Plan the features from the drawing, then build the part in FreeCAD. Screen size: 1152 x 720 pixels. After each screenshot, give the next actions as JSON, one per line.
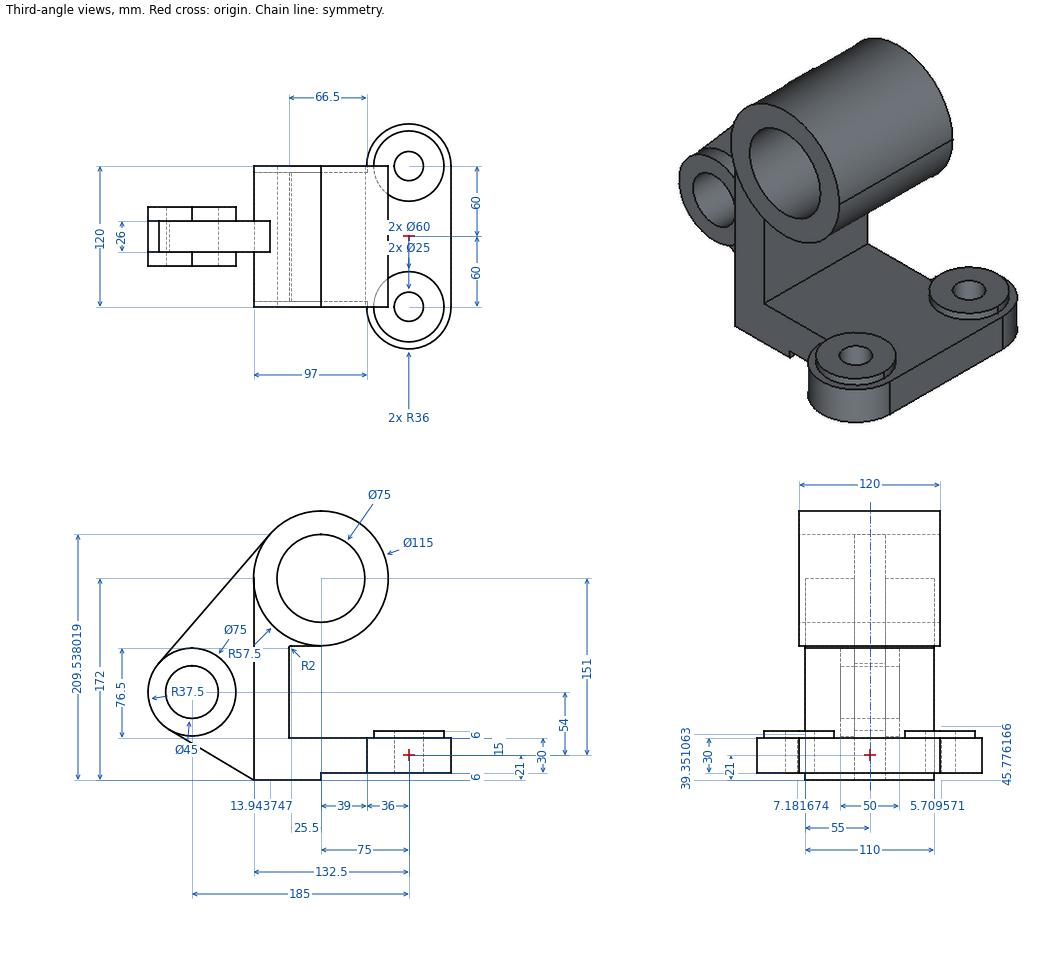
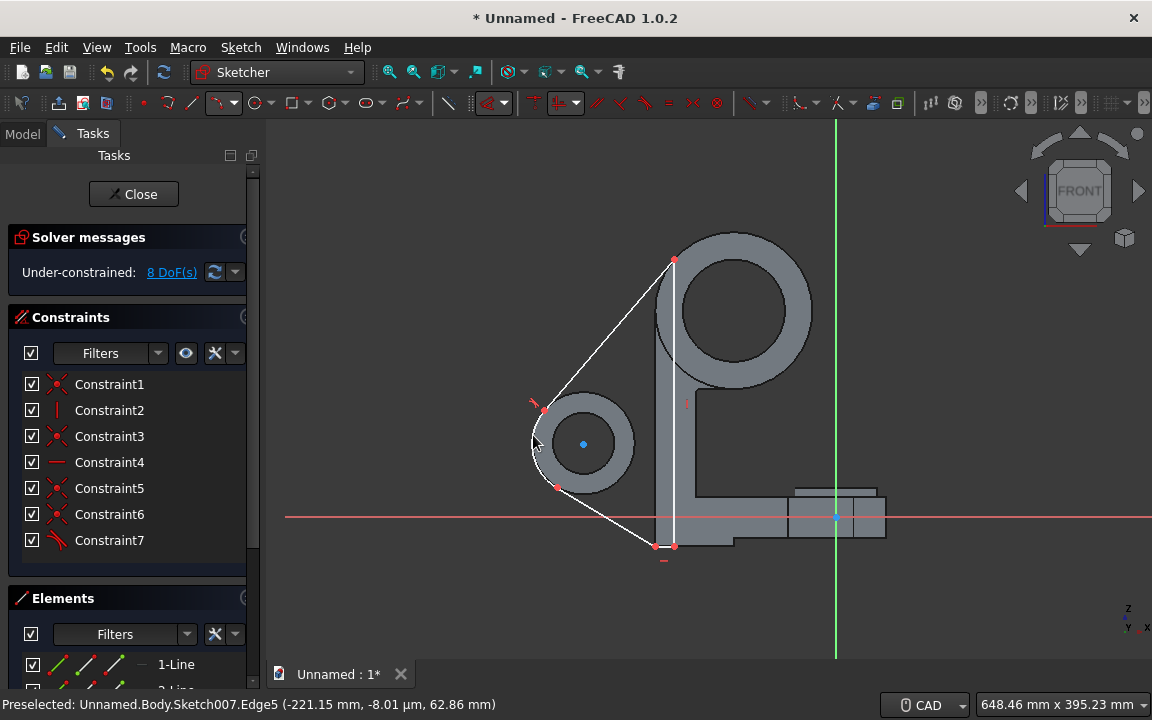
{"action": "left_click", "coordinate": [626, 529]}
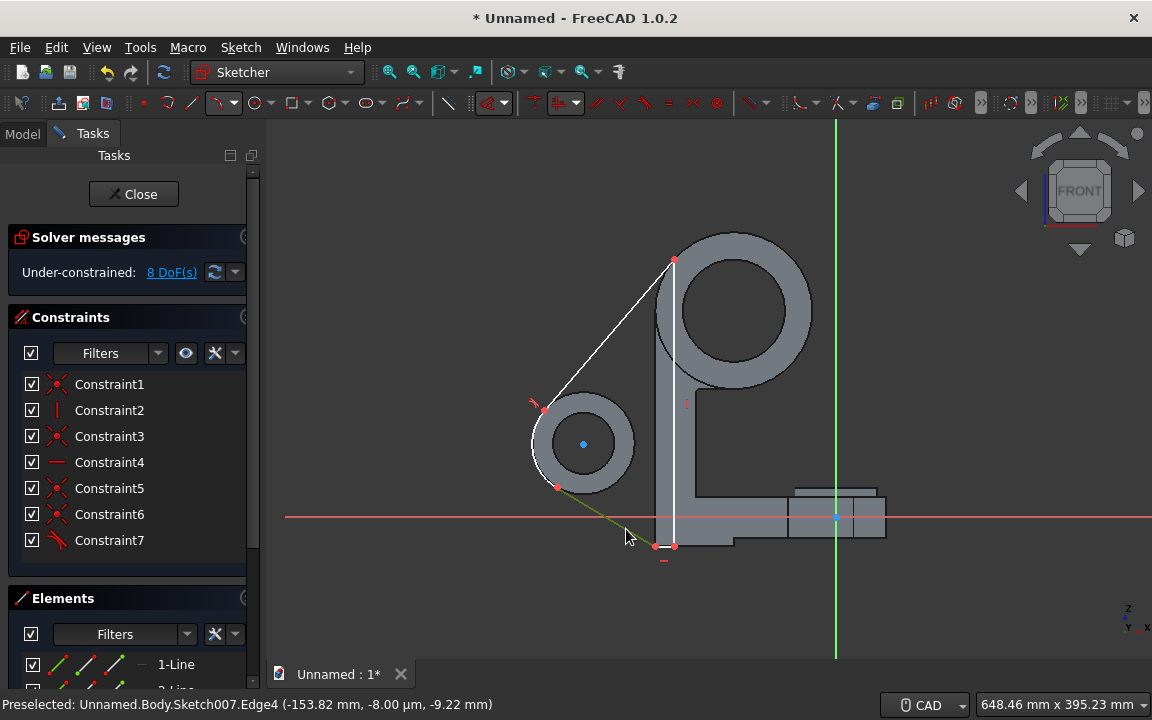
{"action": "left_click", "coordinate": [533, 435]}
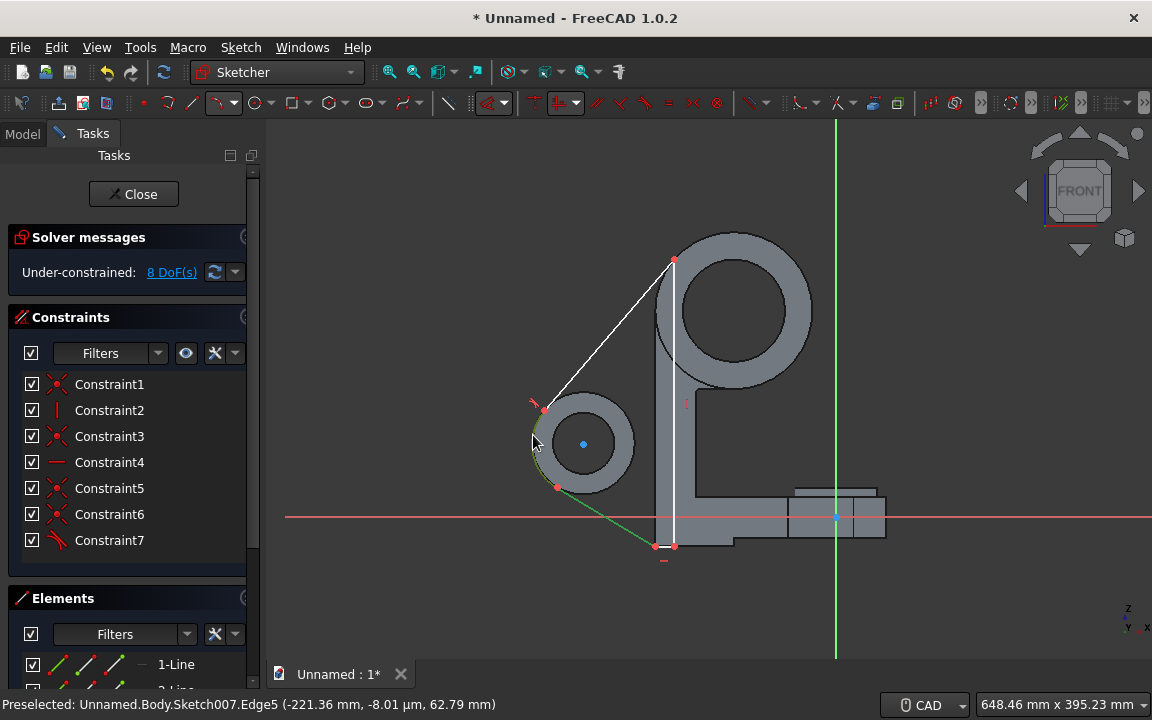
{"action": "left_click", "coordinate": [646, 104]}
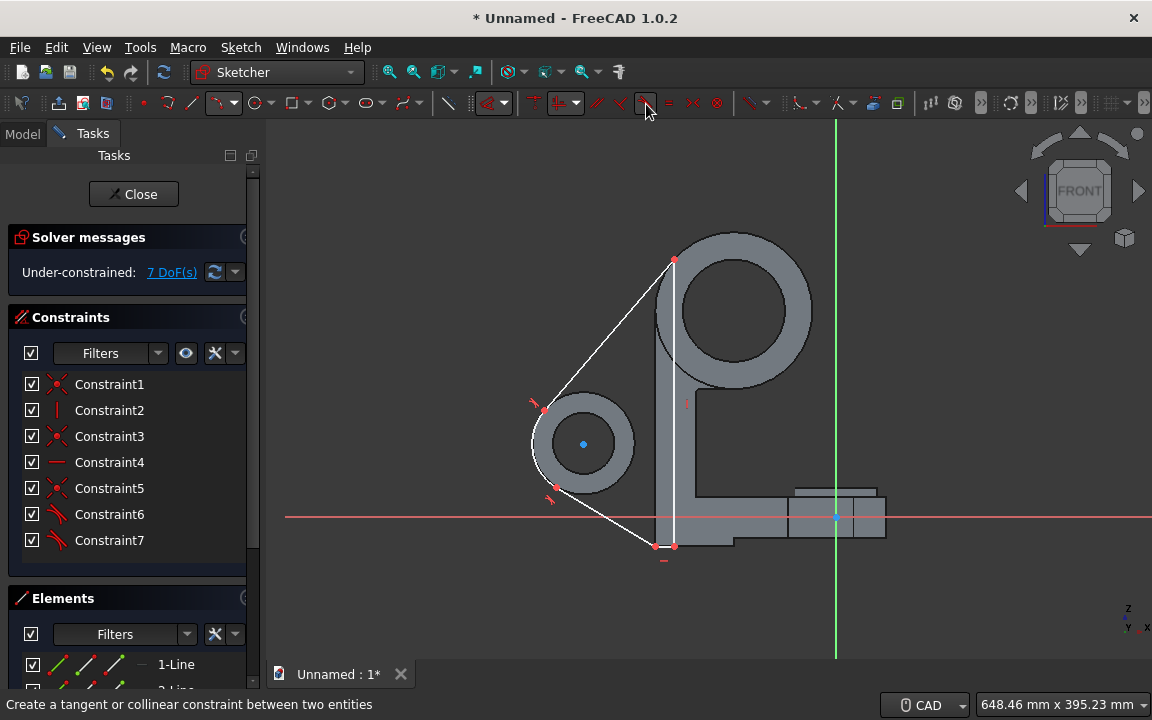
{"action": "left_click", "coordinate": [533, 435]}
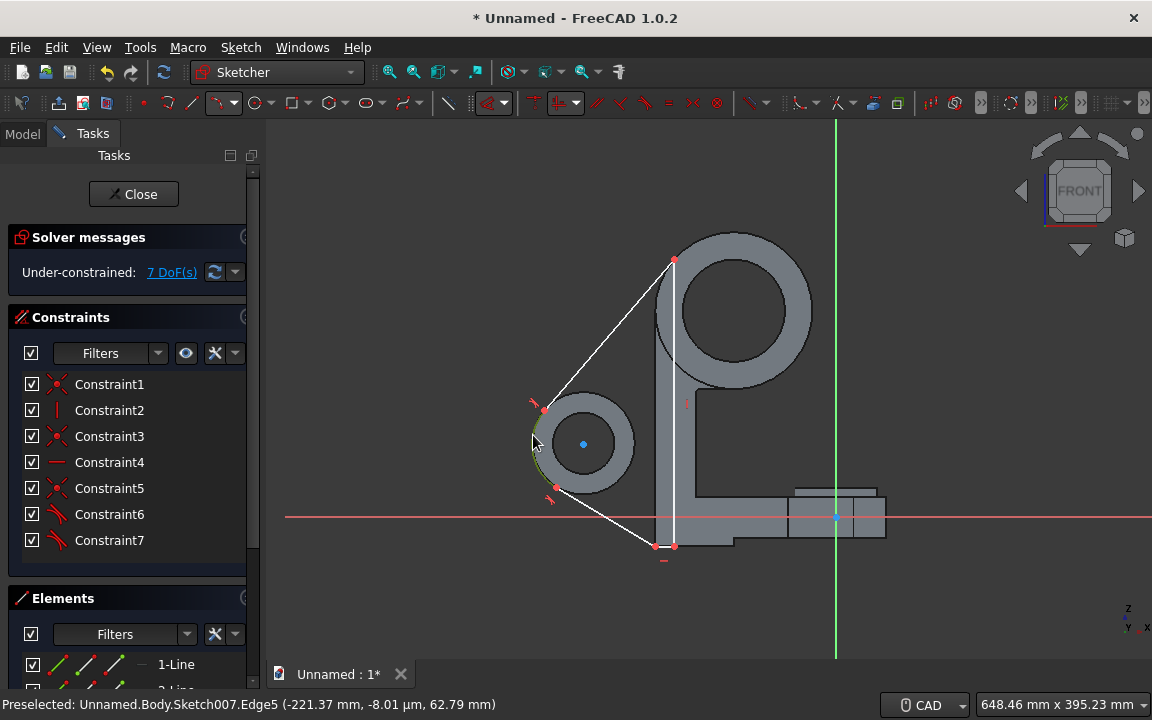
{"action": "key", "text": "k r"}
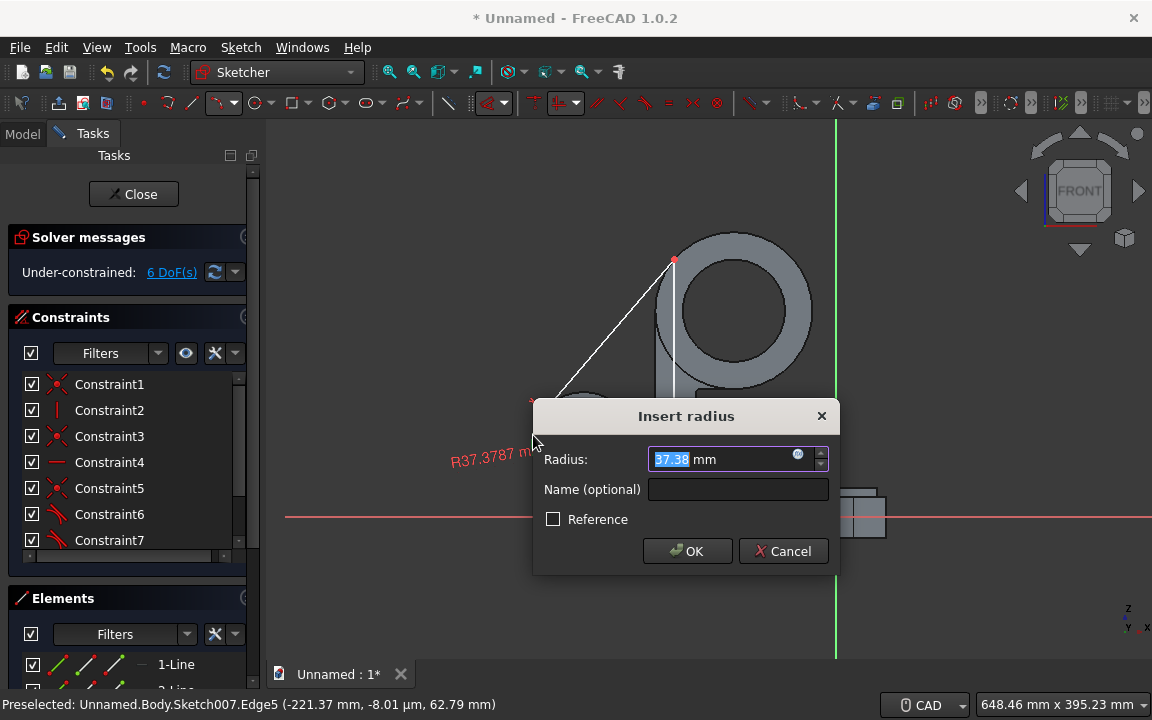
{"action": "type", "text": "37.5"}
{"action": "key", "text": "Return"}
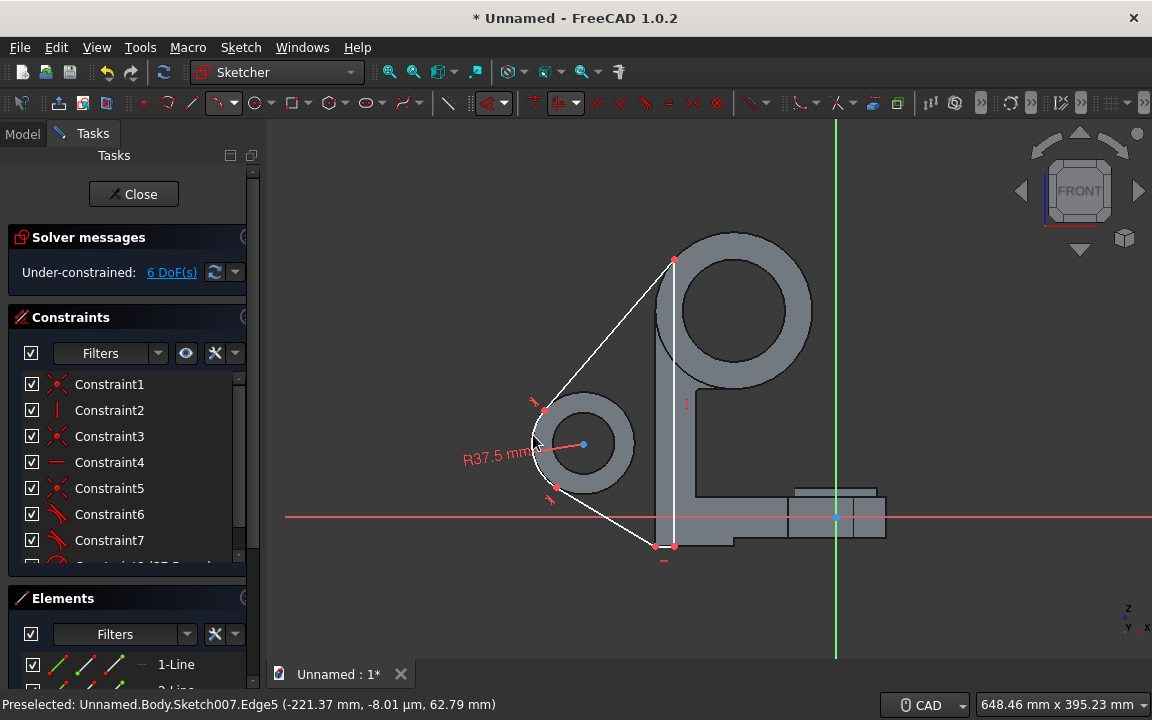
{"action": "scroll", "coordinate": [674, 547], "scroll_direction": "up", "scroll_amount": 2}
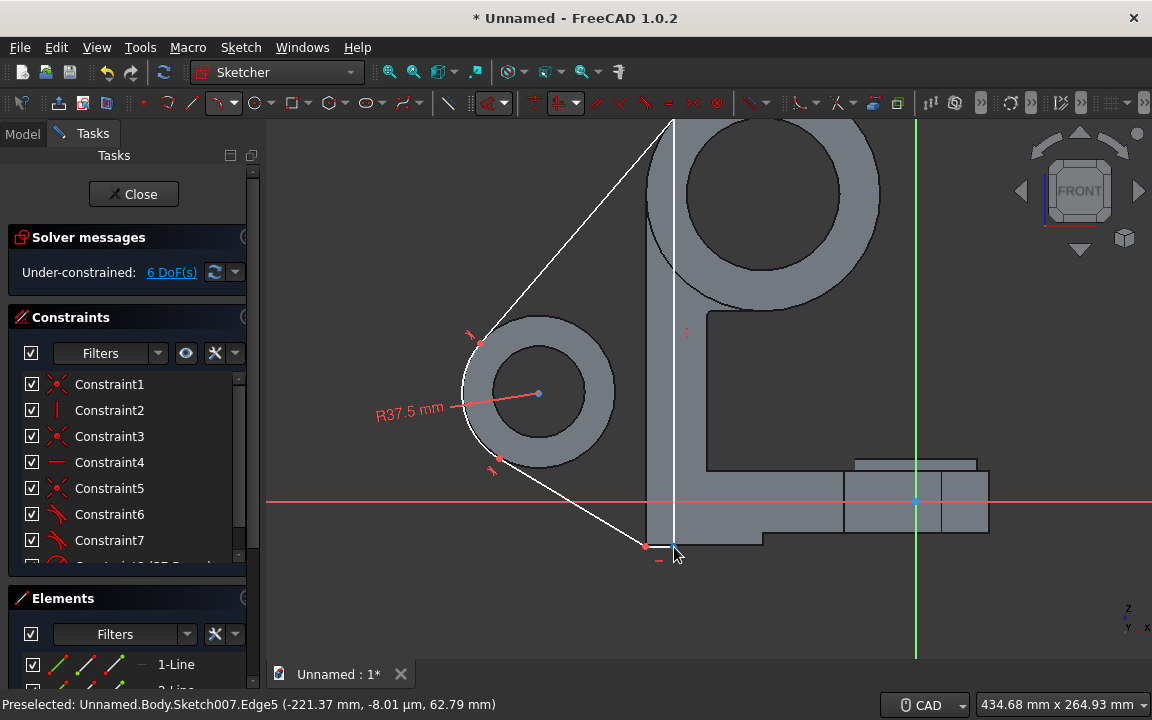
{"action": "left_click", "coordinate": [674, 547]}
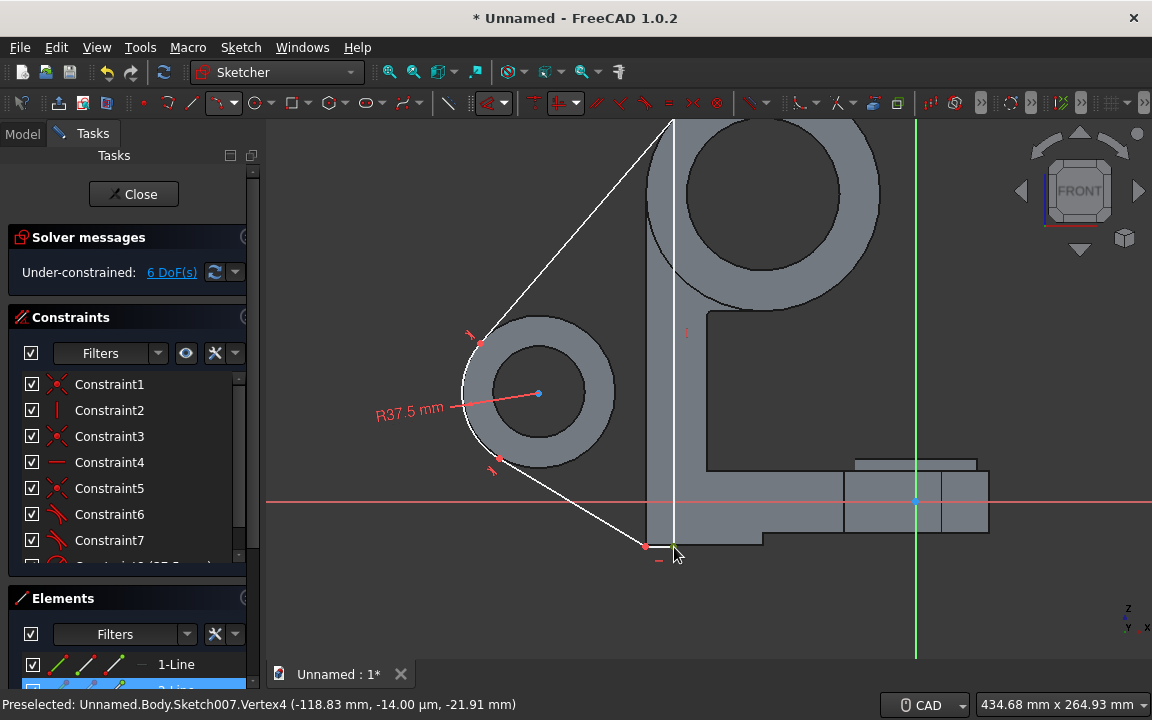
{"action": "left_click", "coordinate": [506, 104]}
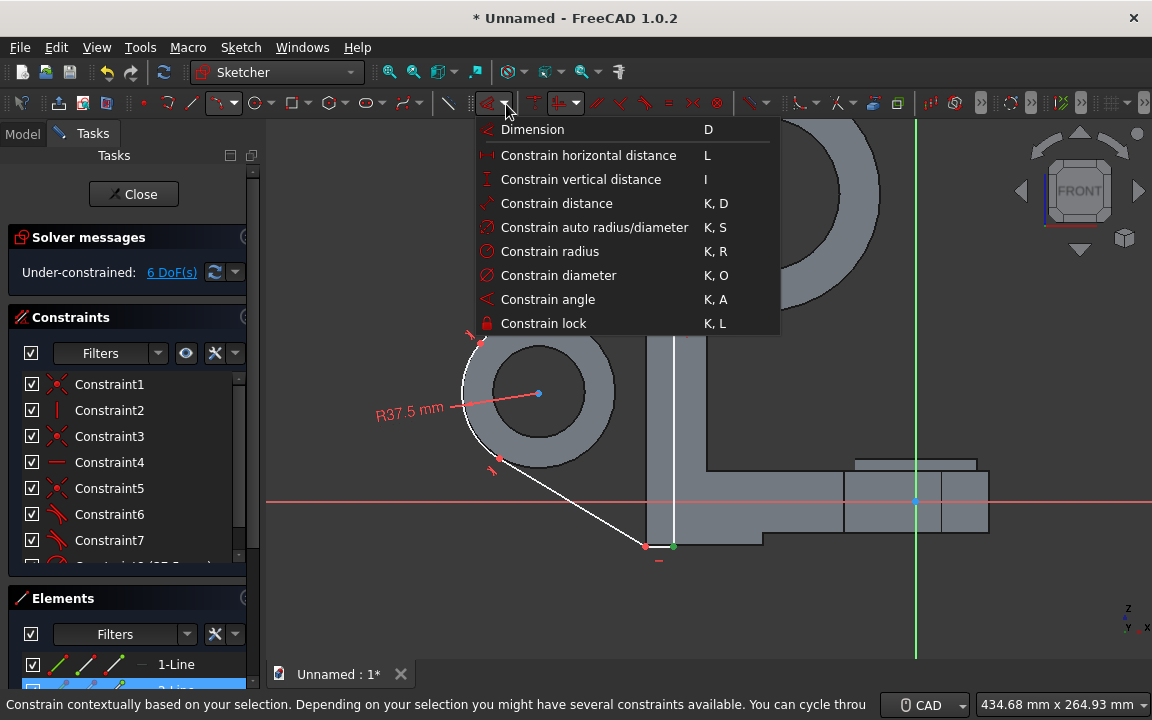
{"action": "left_click", "coordinate": [628, 179]}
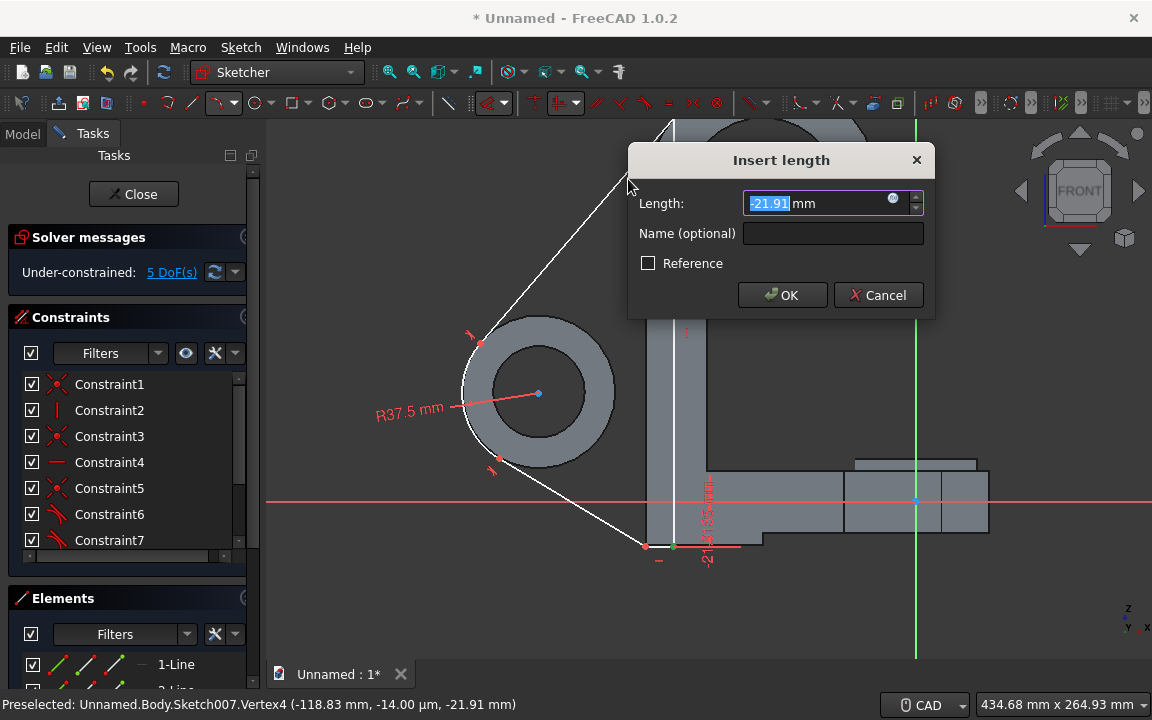
{"action": "type", "text": "-21"}
{"action": "key", "text": "Return"}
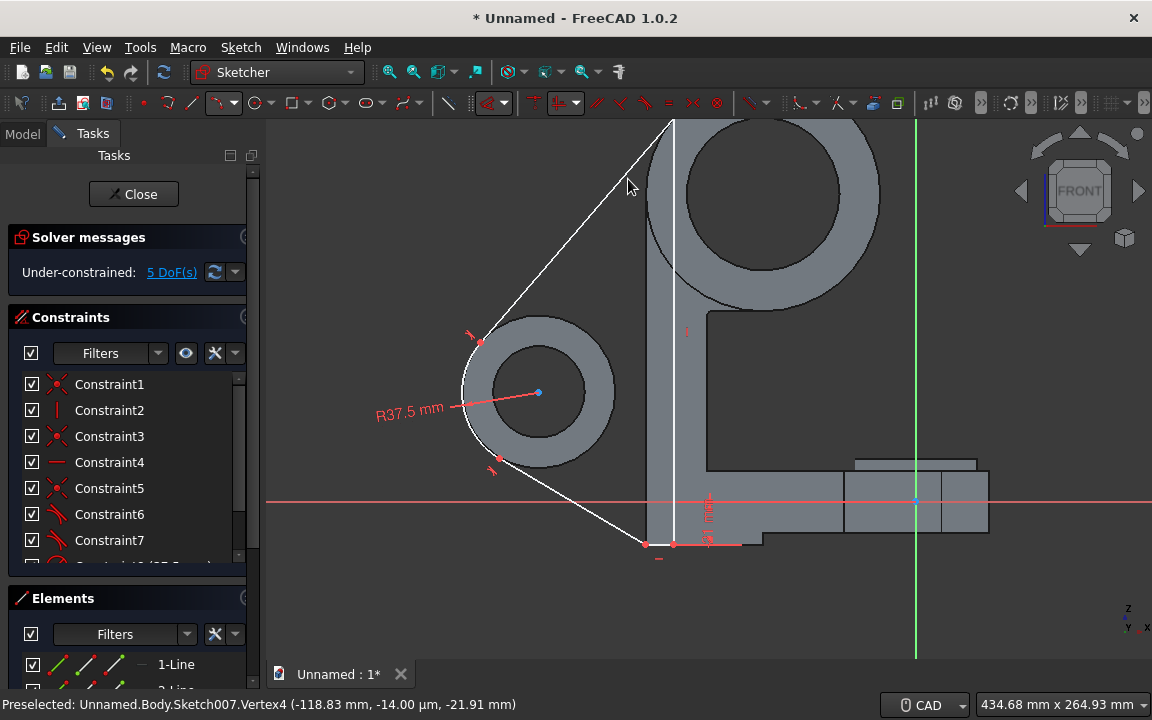
{"action": "left_click", "coordinate": [539, 393]}